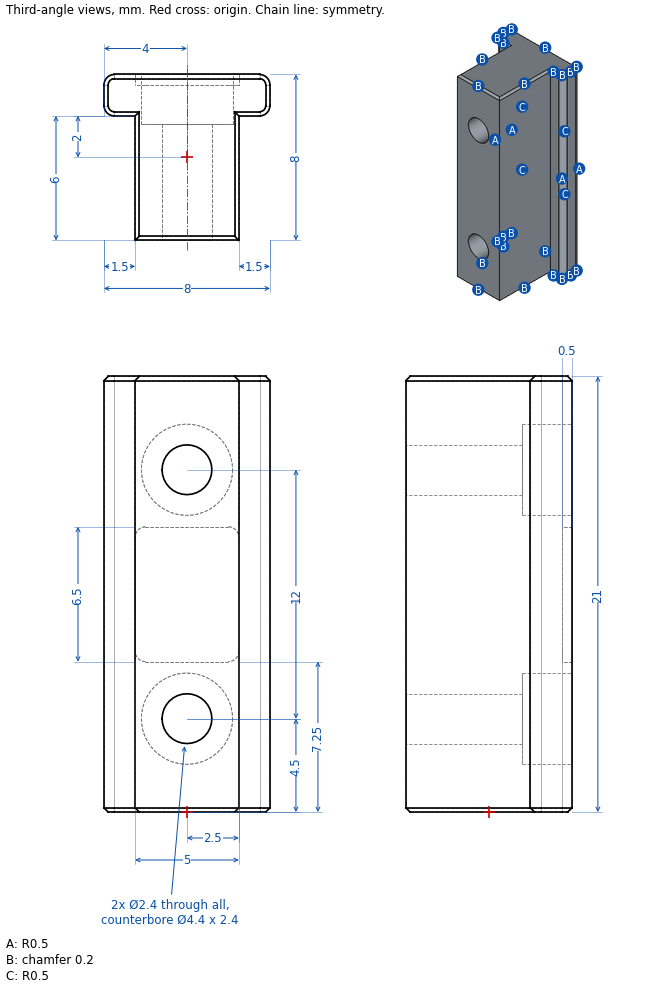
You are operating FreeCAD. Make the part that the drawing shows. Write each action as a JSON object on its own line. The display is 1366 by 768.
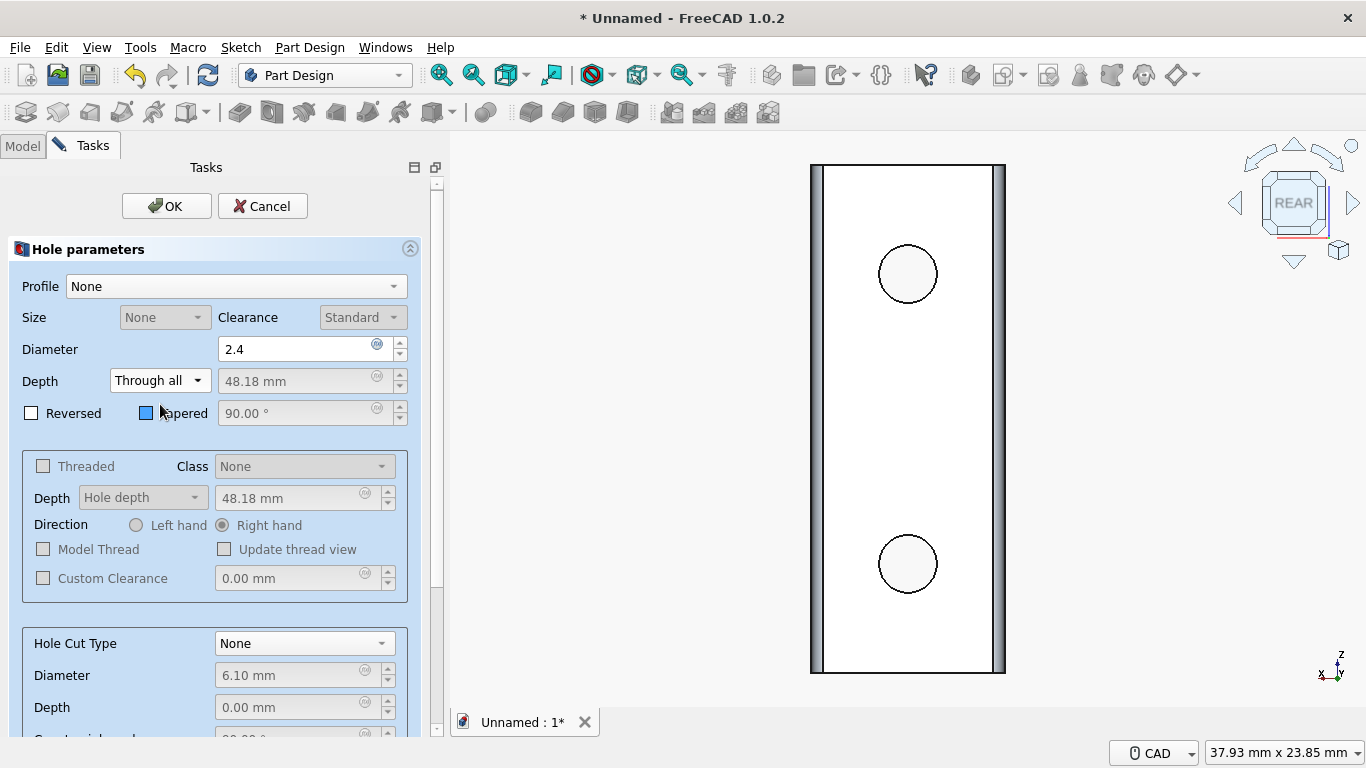
{"action": "left_click", "coordinate": [306, 644]}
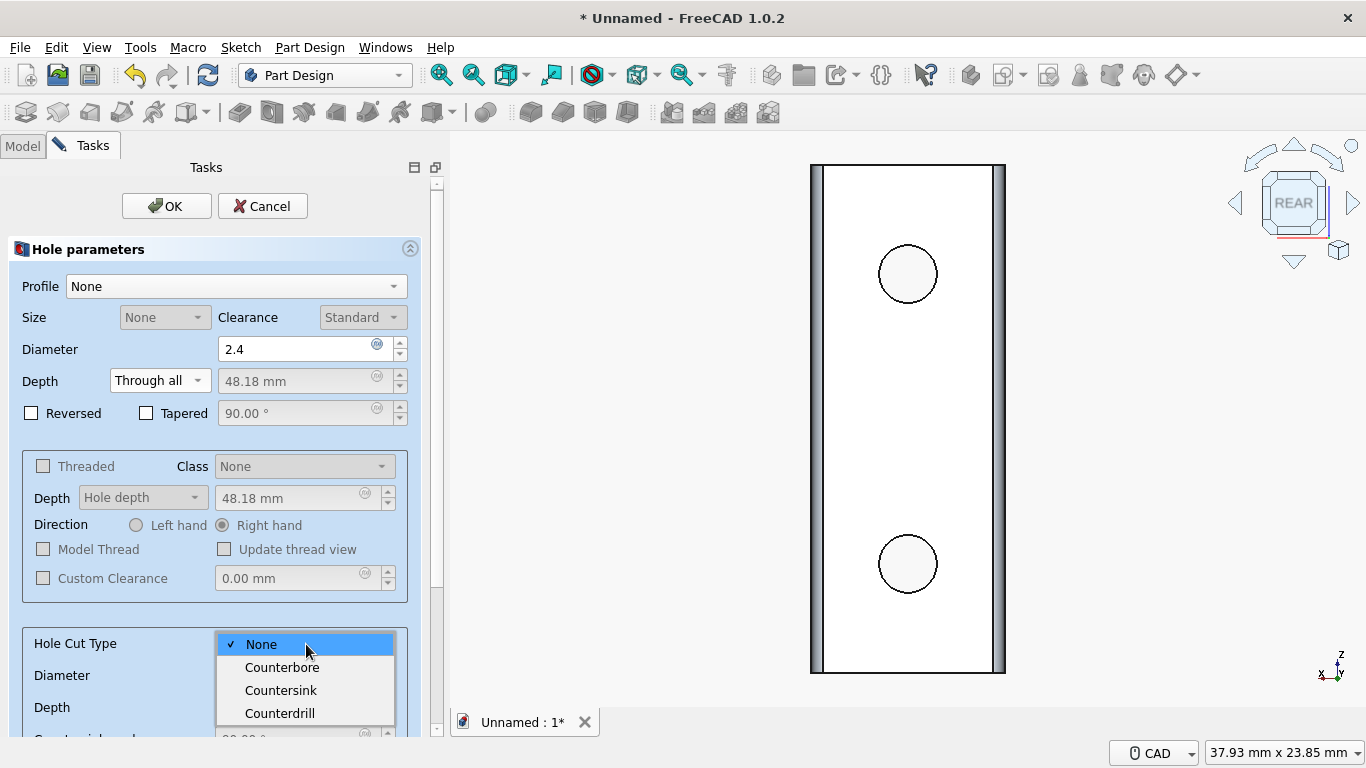
{"action": "left_click", "coordinate": [304, 668]}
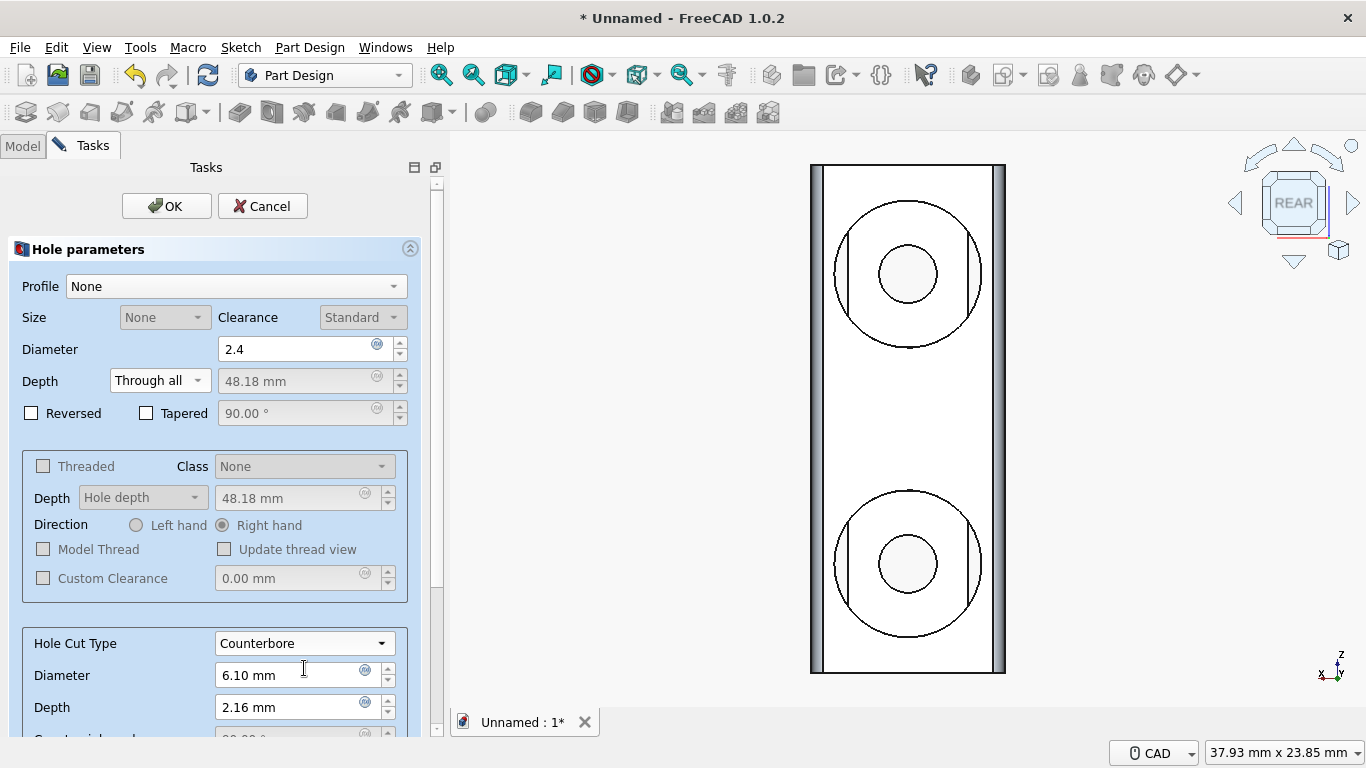
{"action": "triple_click", "coordinate": [298, 675]}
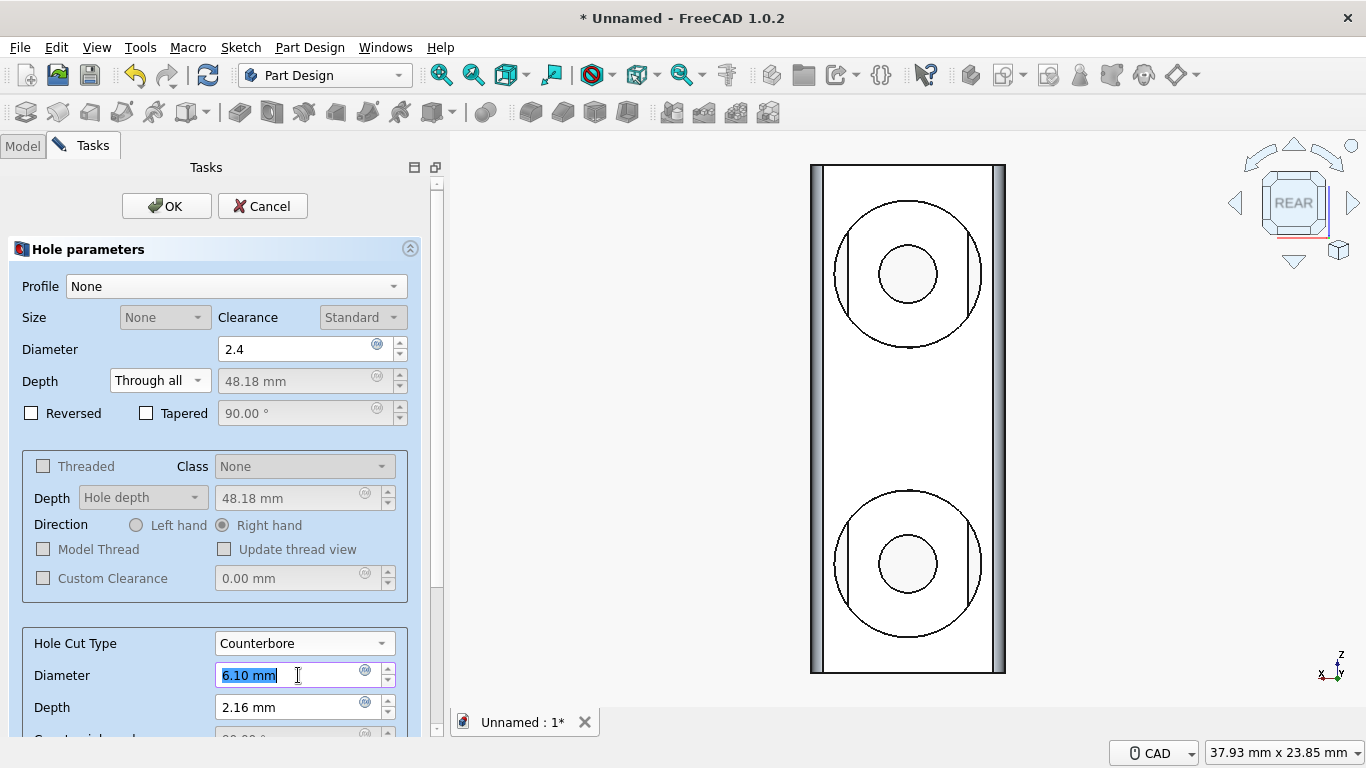
{"action": "type", "text": "4.4"}
{"action": "key", "text": "Tab"}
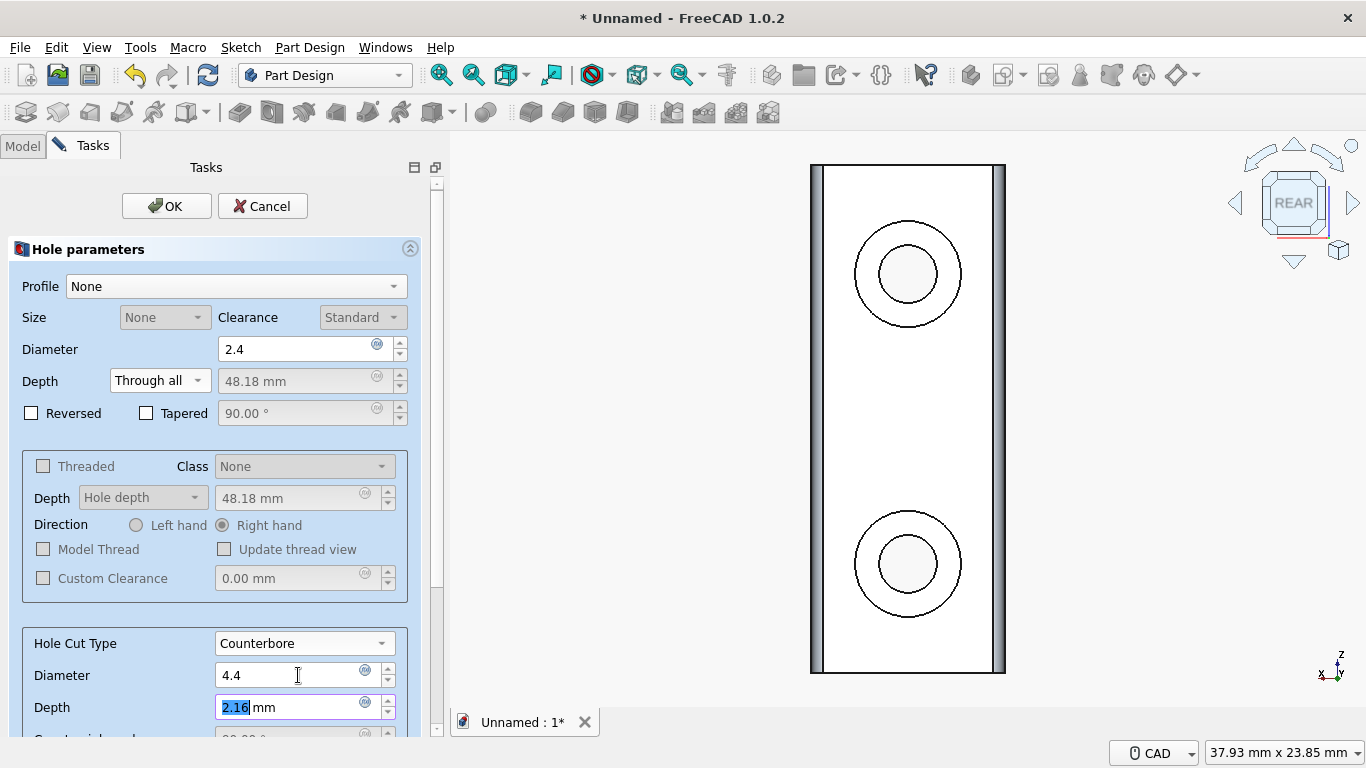
{"action": "type", "text": "2.4"}
{"action": "key", "text": "Tab"}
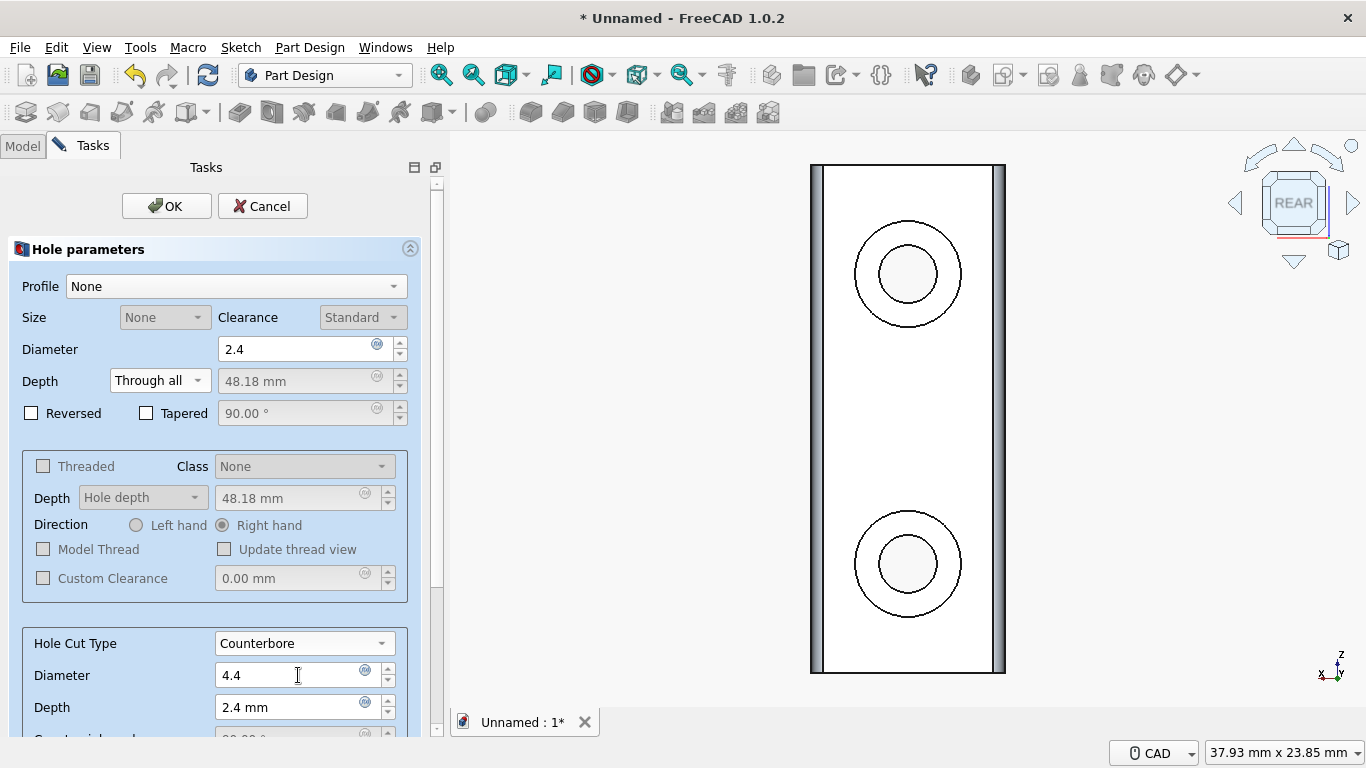
{"action": "left_click", "coordinate": [167, 206]}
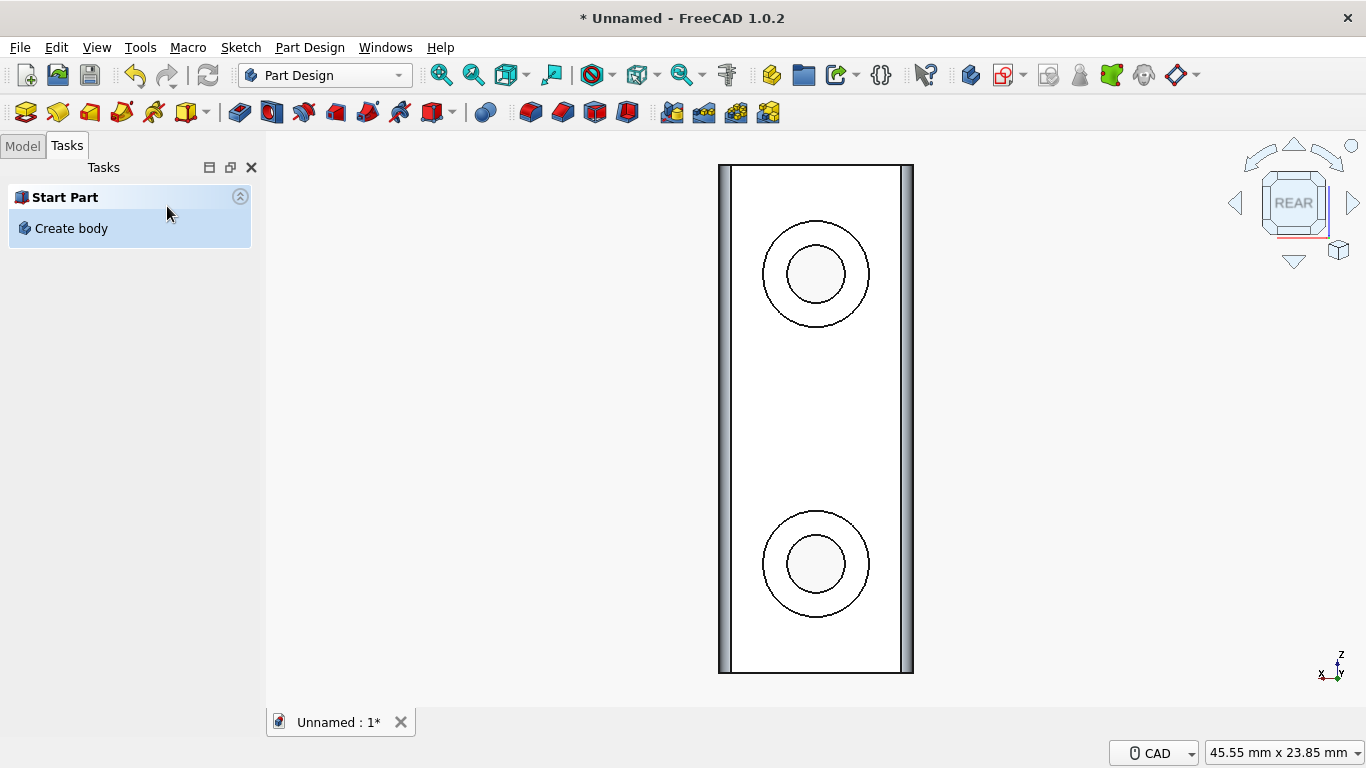
{"action": "key", "text": "0"}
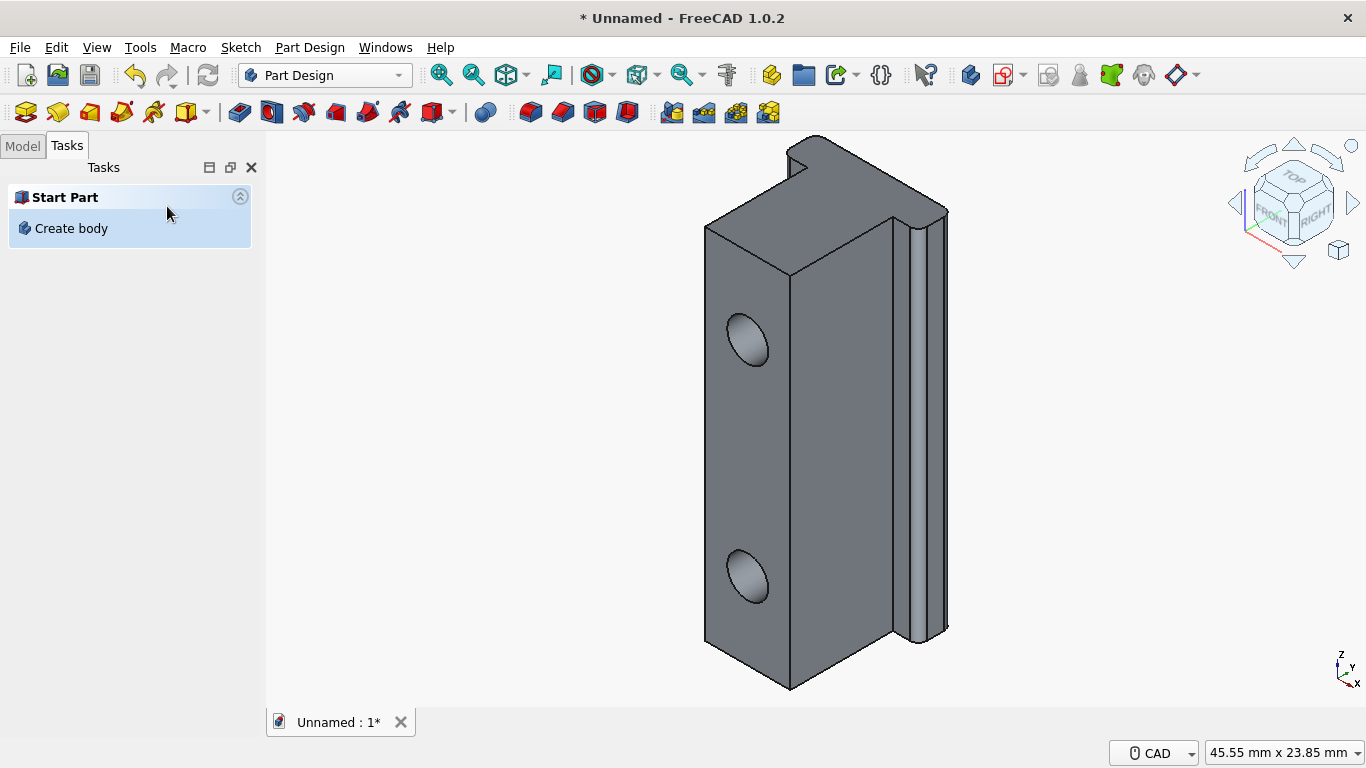
{"action": "left_click", "coordinate": [836, 200]}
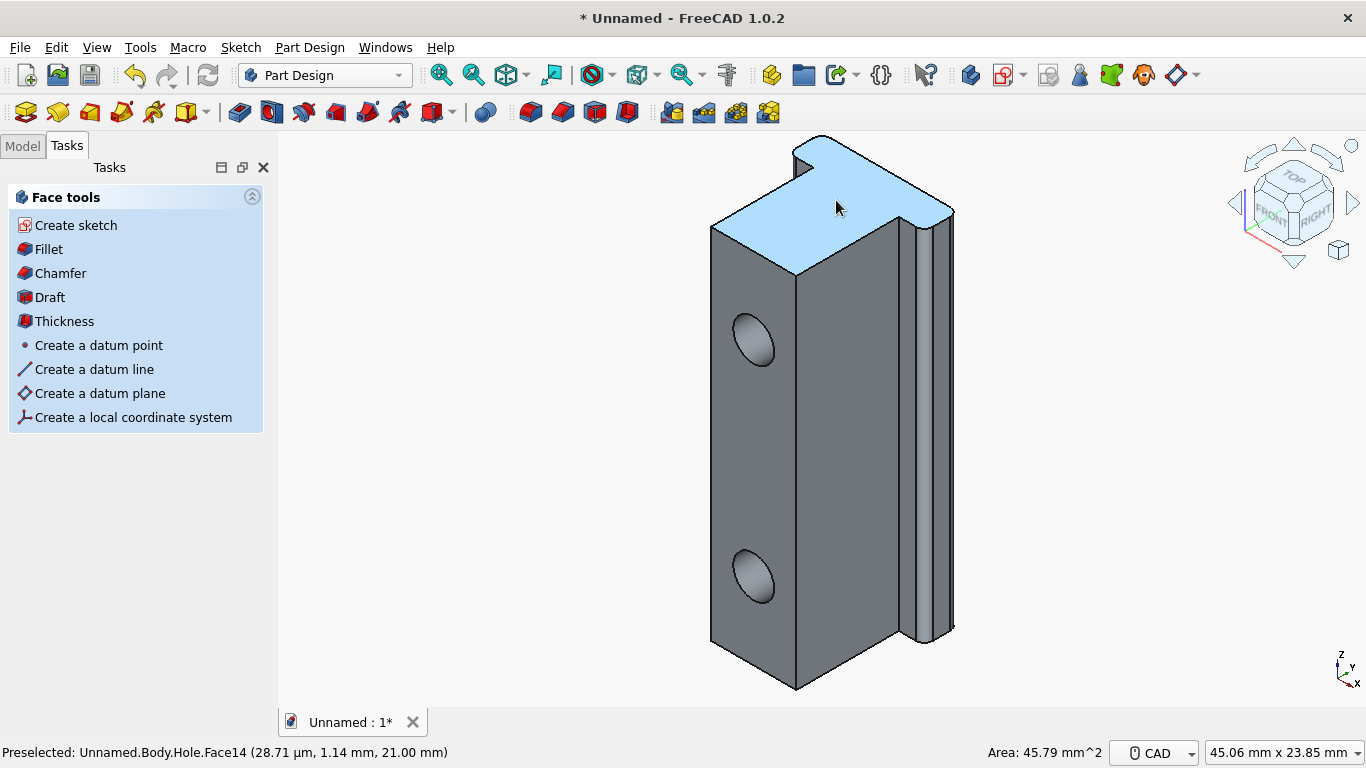
{"action": "key", "text": "2"}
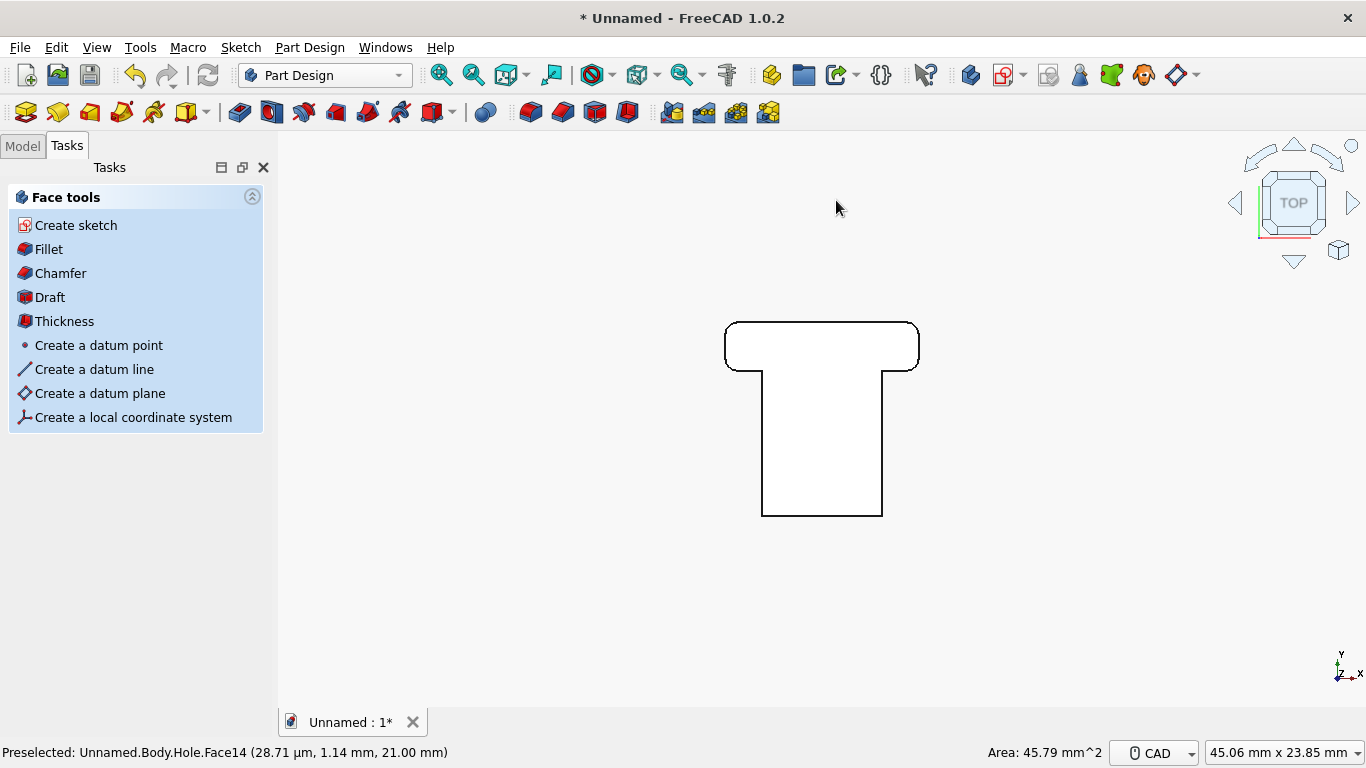
{"action": "left_click", "coordinate": [442, 76]}